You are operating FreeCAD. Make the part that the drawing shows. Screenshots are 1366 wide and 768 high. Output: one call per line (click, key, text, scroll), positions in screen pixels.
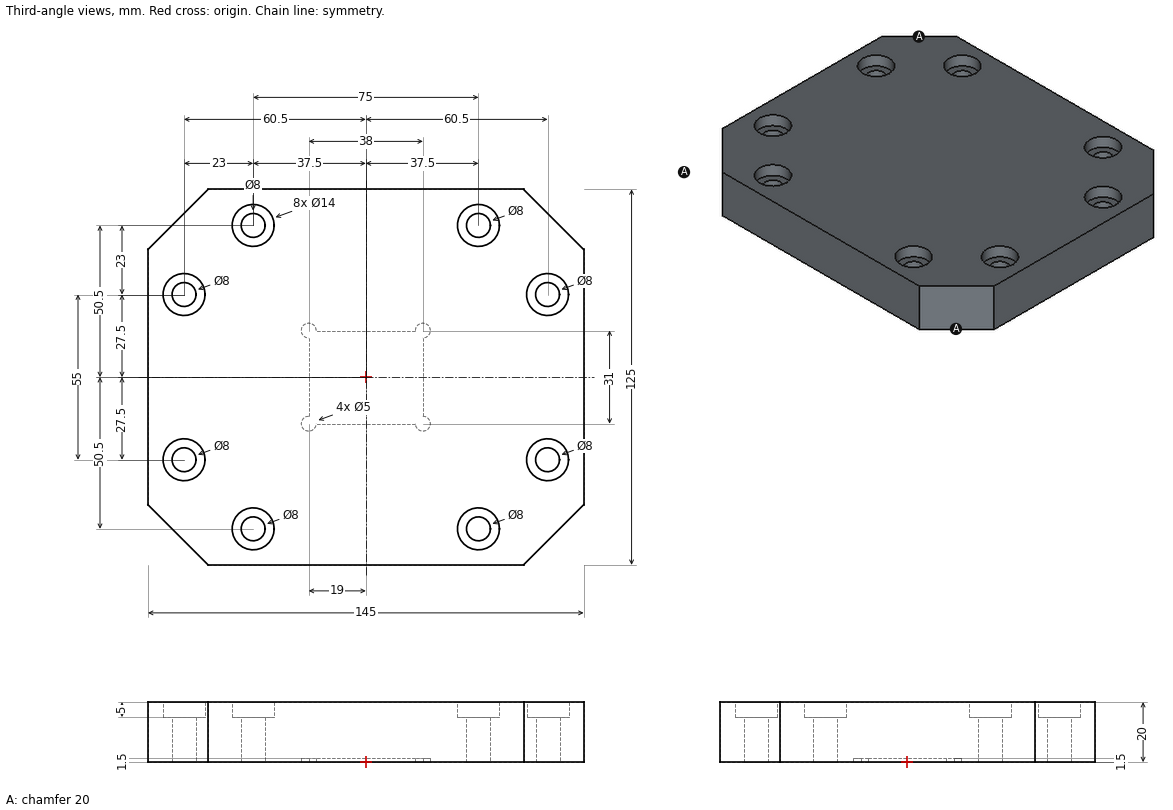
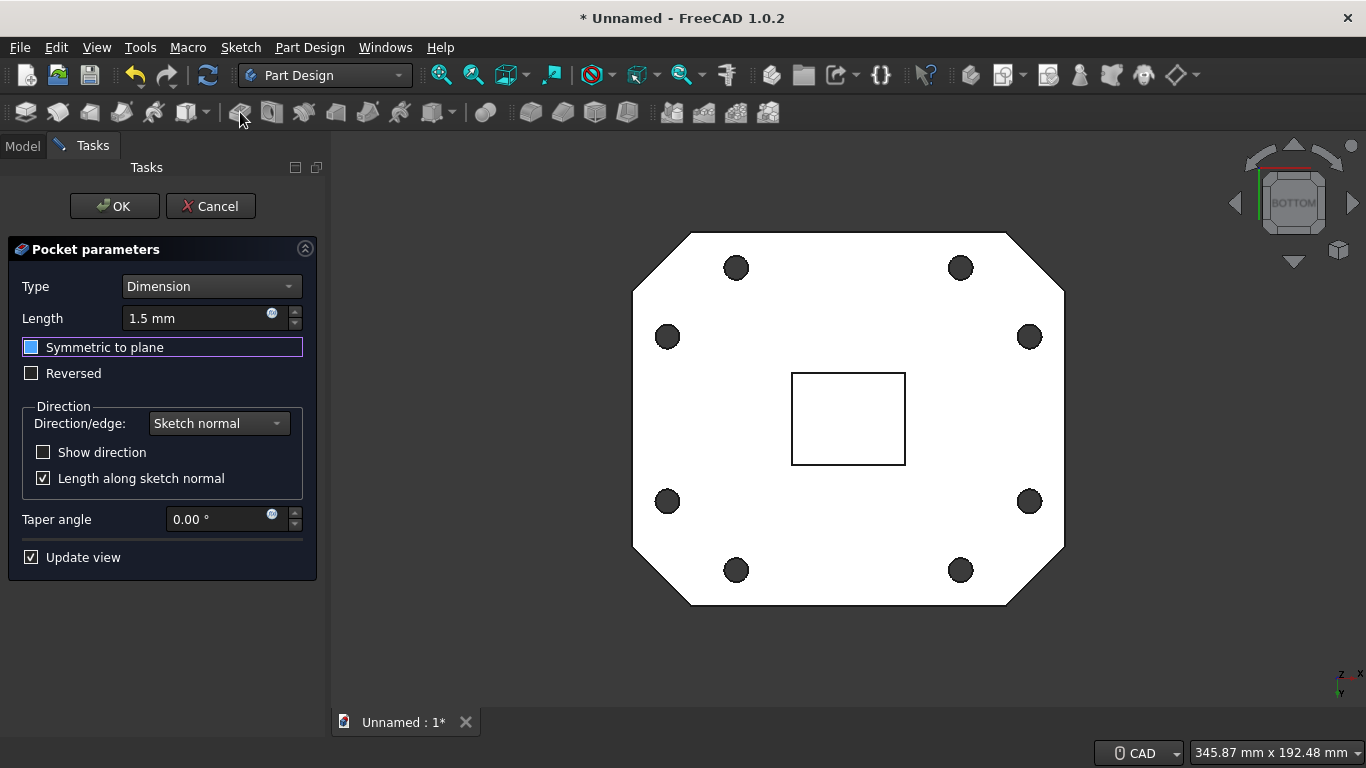
click(115, 206)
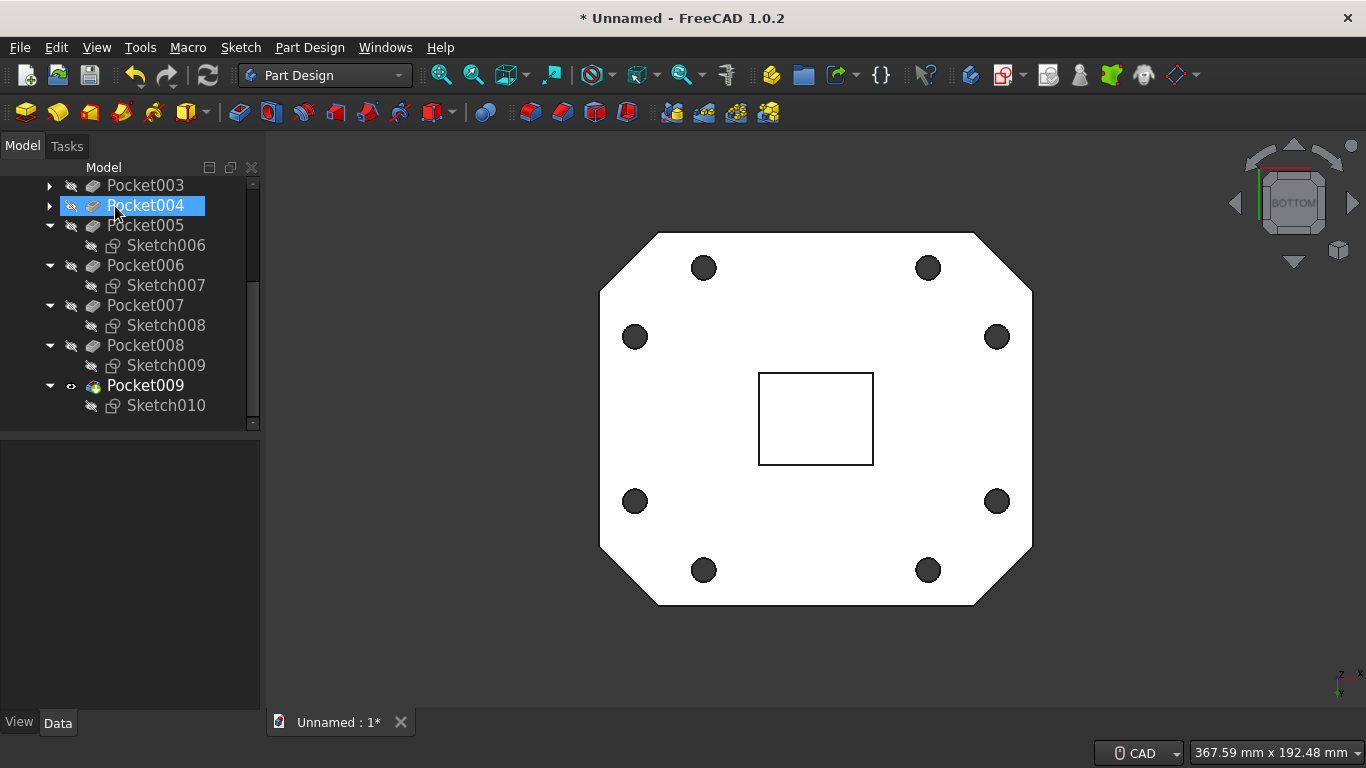
click(940, 418)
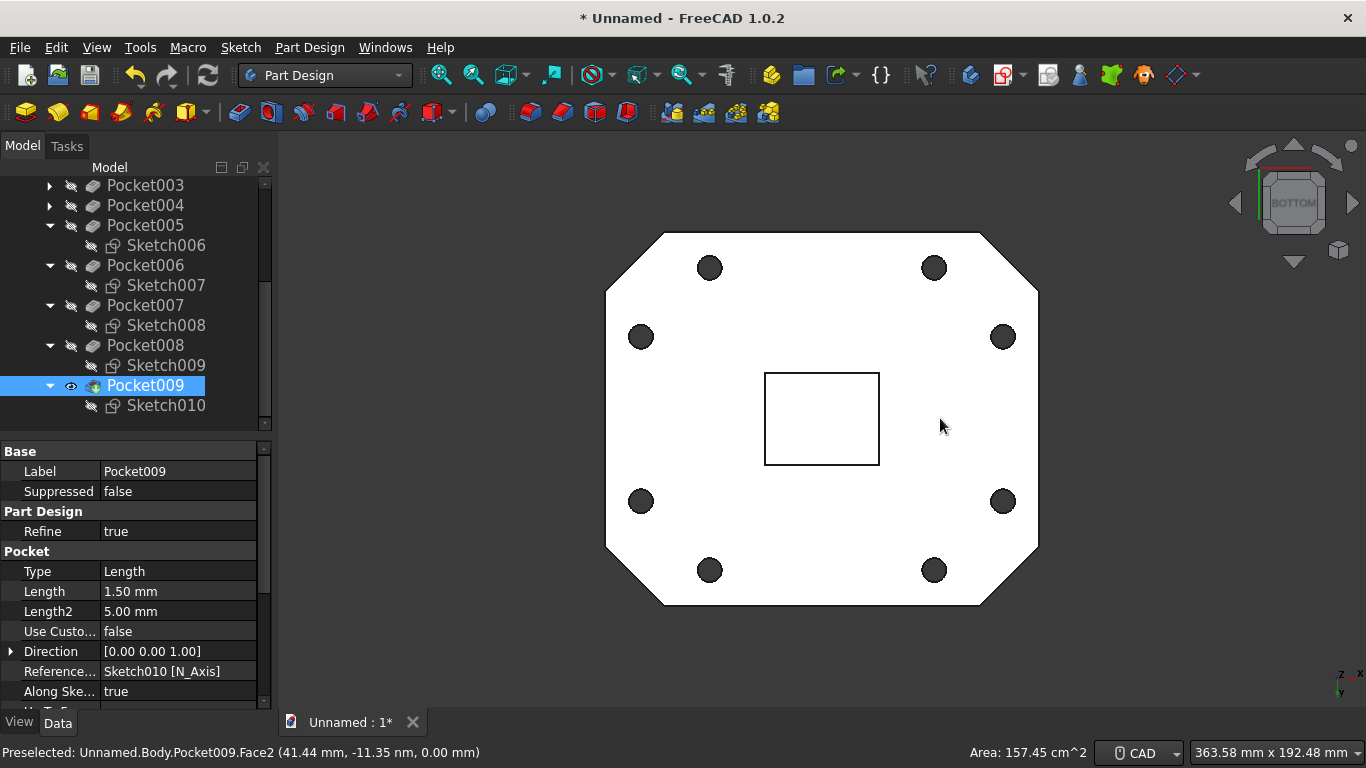
click(1004, 76)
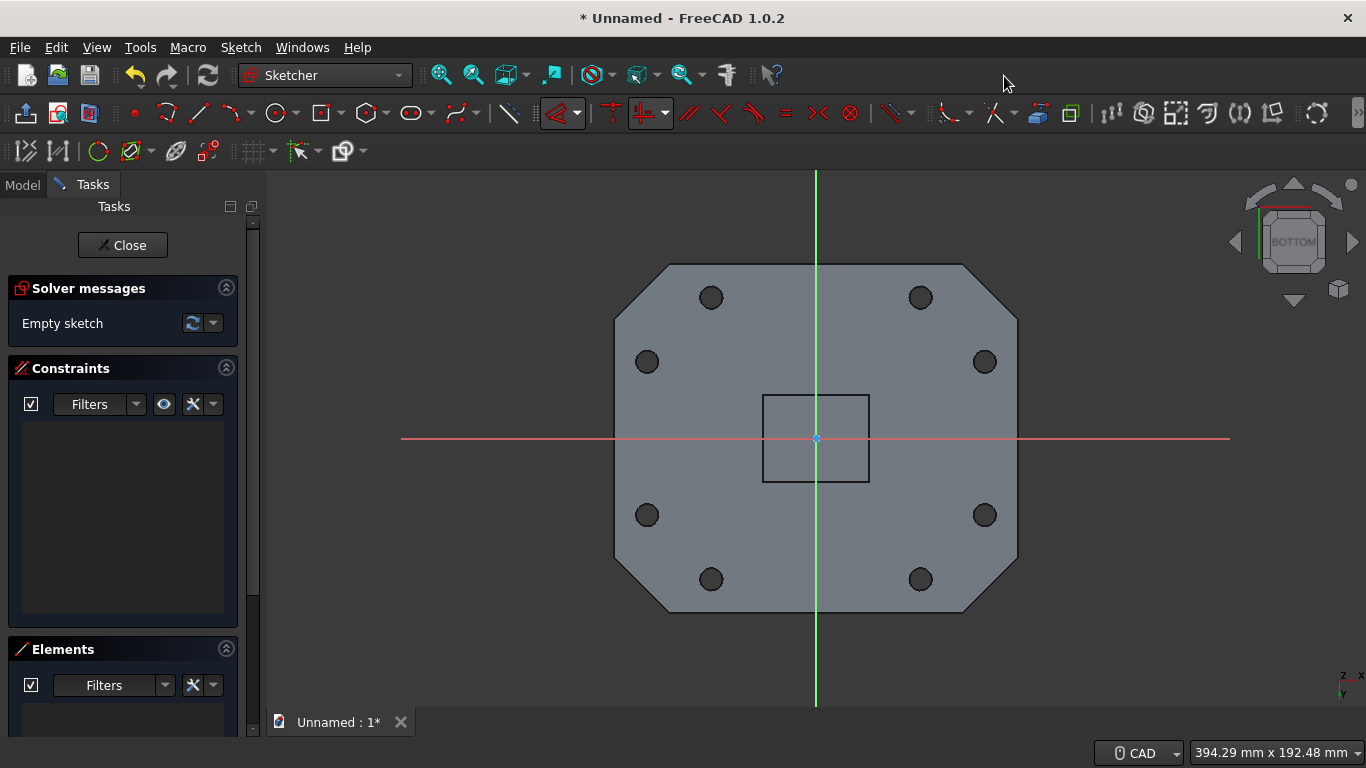
scroll(846, 439, up, 6)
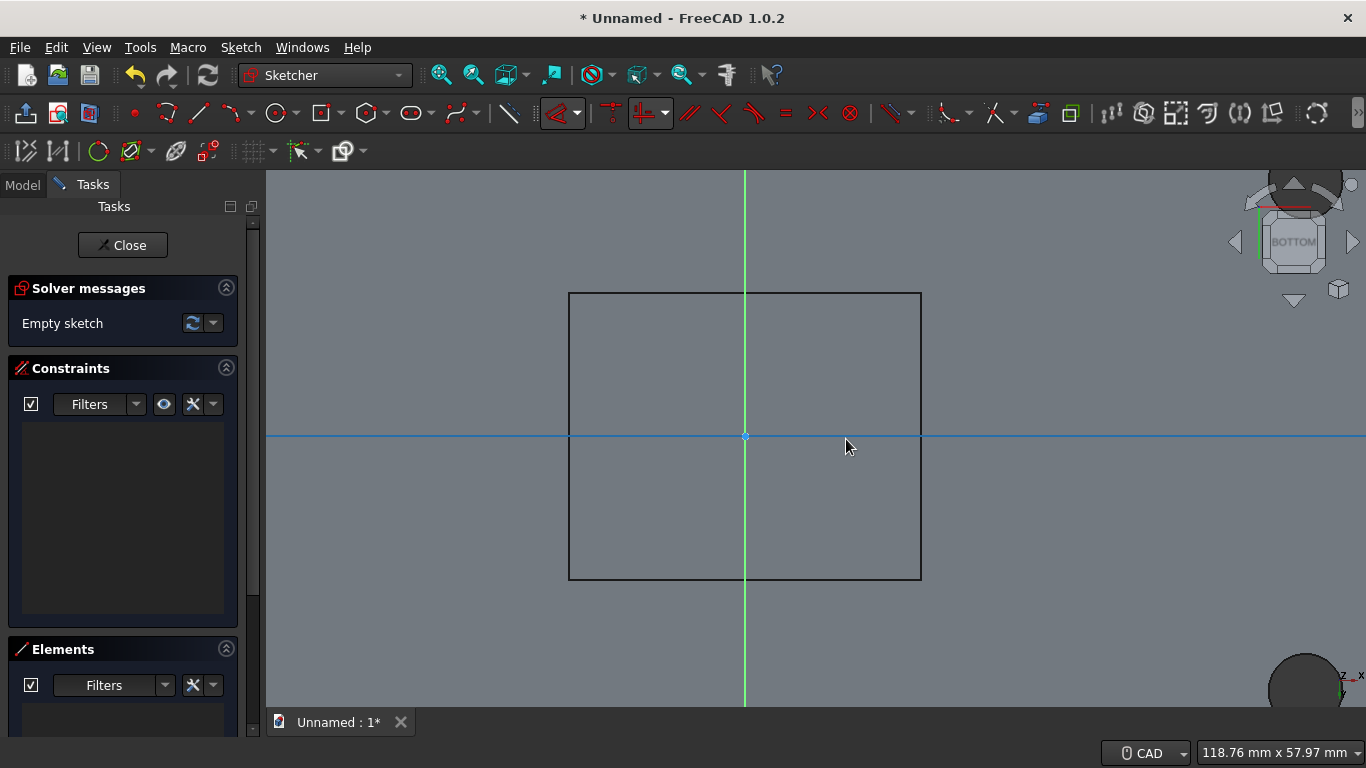
click(276, 114)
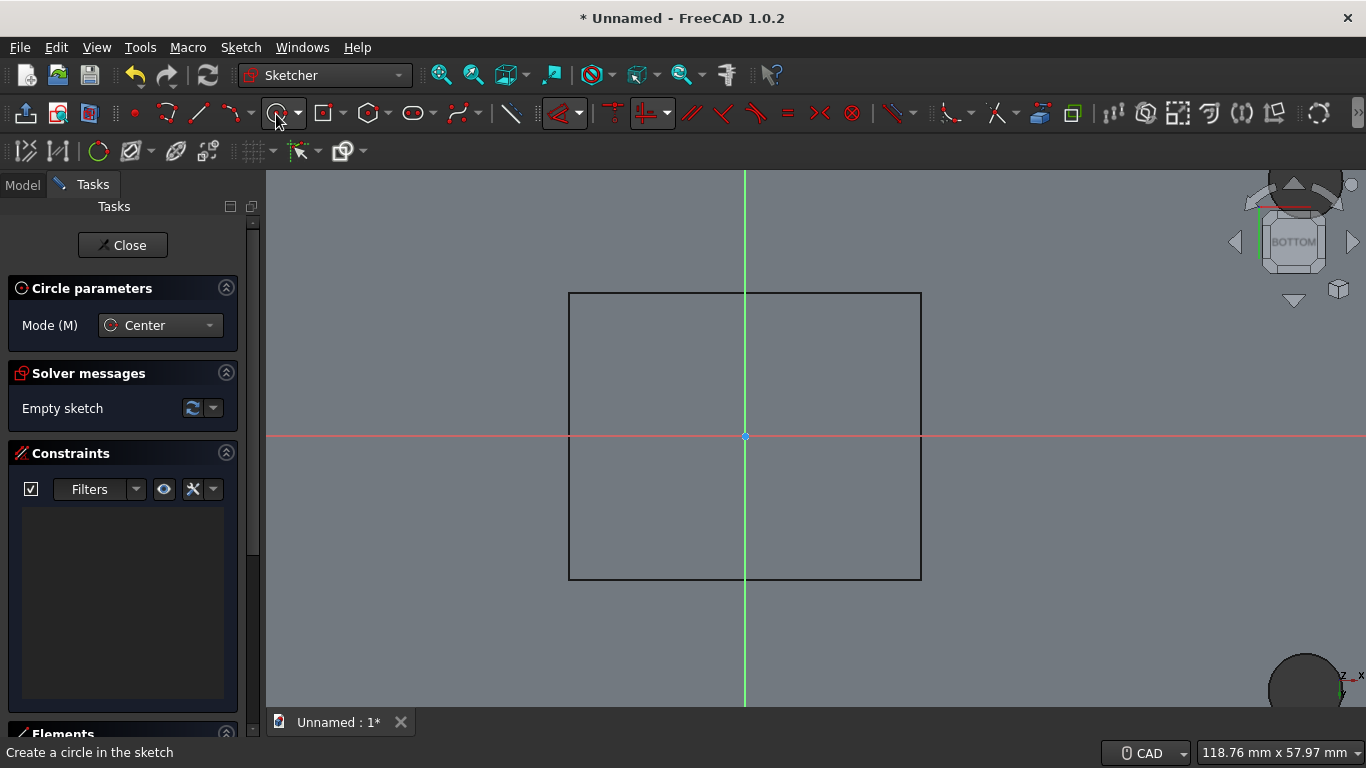
click(569, 293)
click(586, 276)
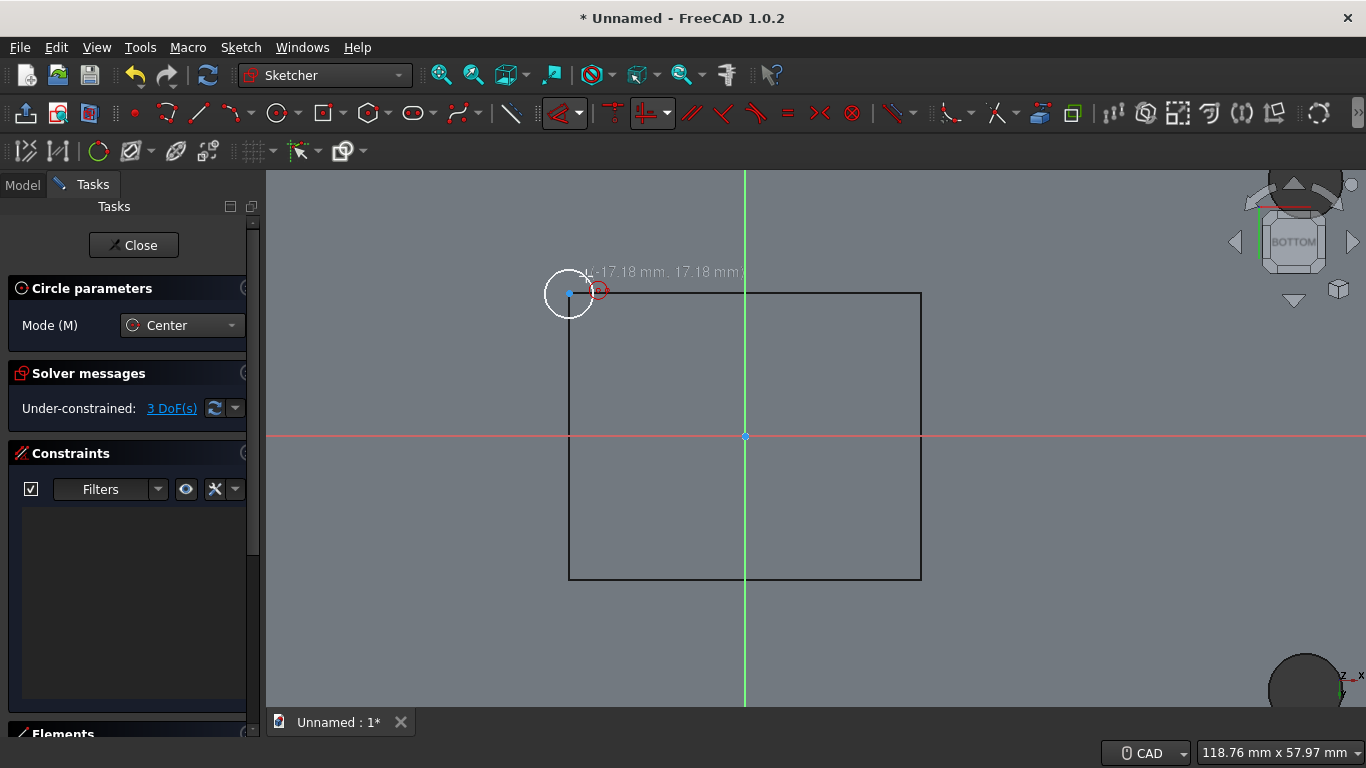
click(921, 293)
click(938, 276)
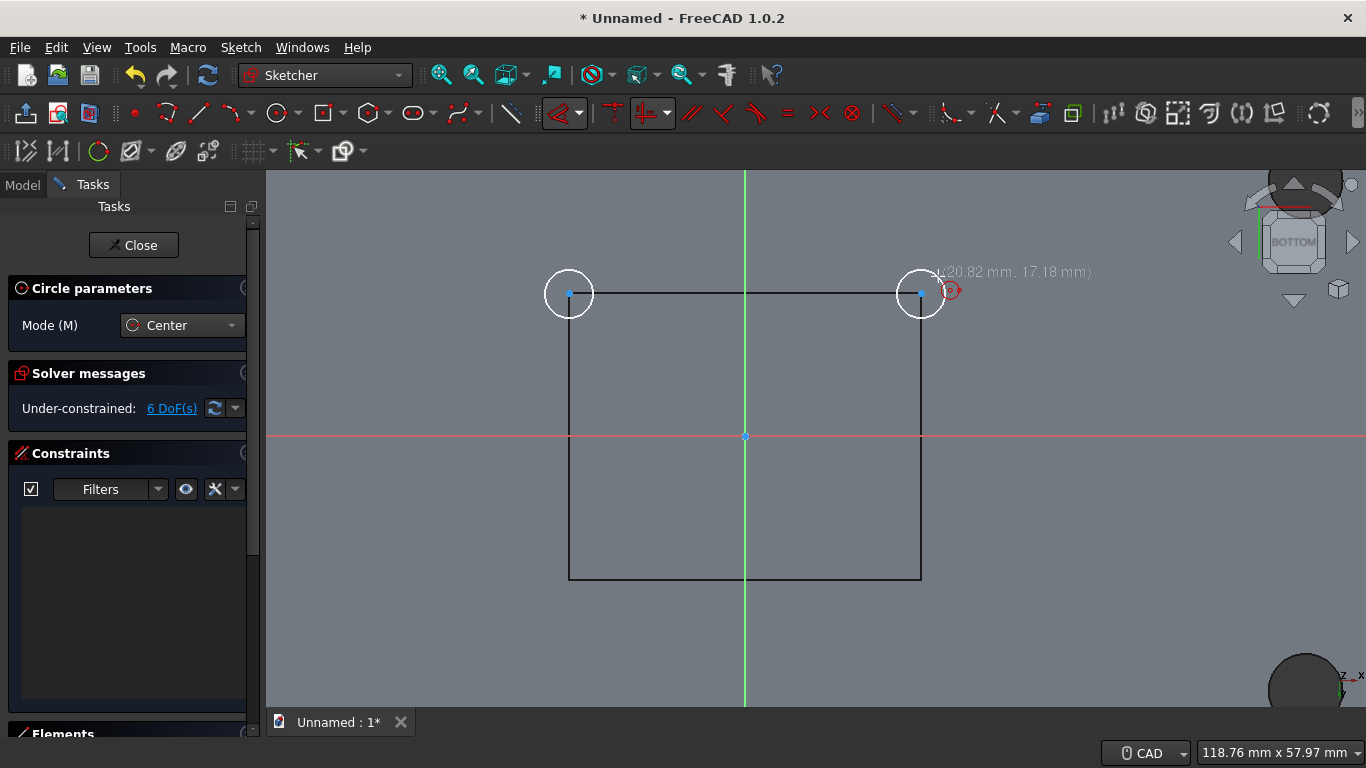
click(921, 580)
click(938, 563)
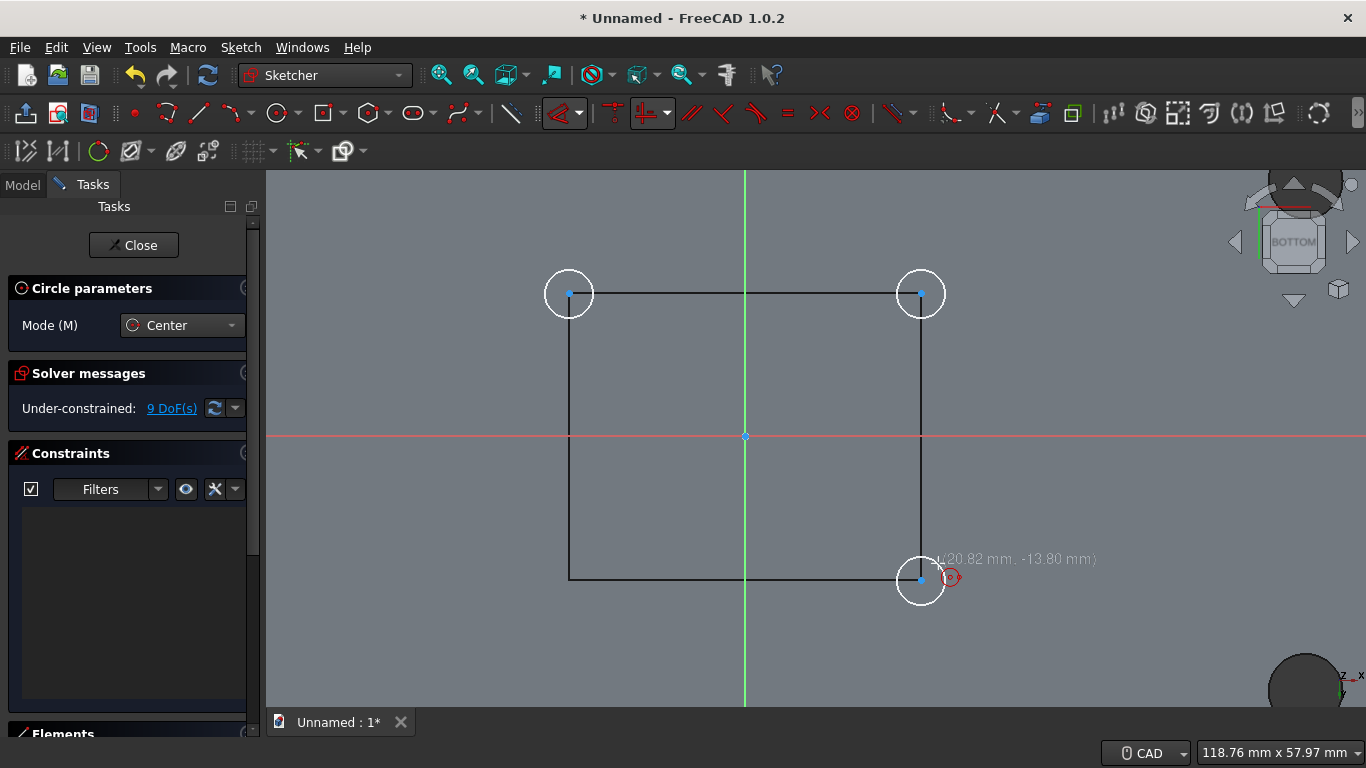
click(569, 580)
click(586, 563)
key(Escape)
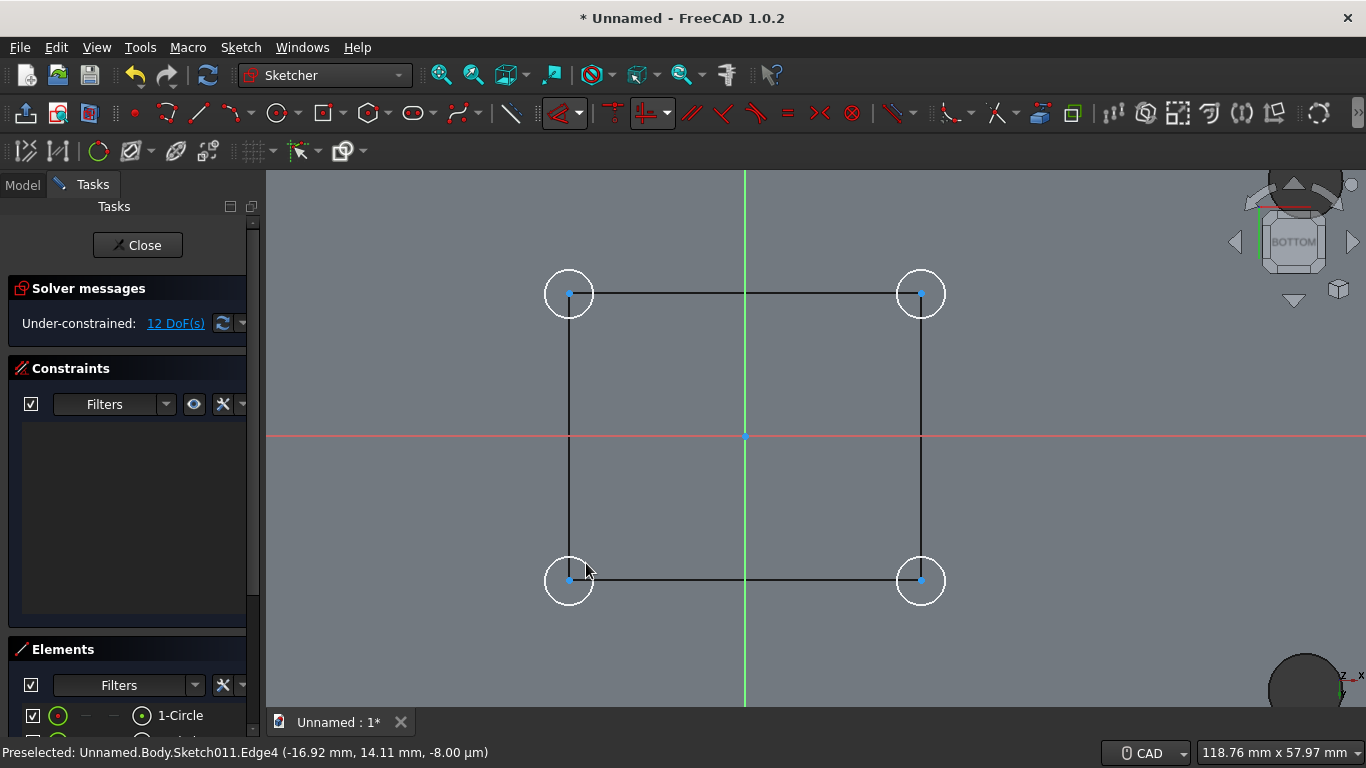
click(586, 277)